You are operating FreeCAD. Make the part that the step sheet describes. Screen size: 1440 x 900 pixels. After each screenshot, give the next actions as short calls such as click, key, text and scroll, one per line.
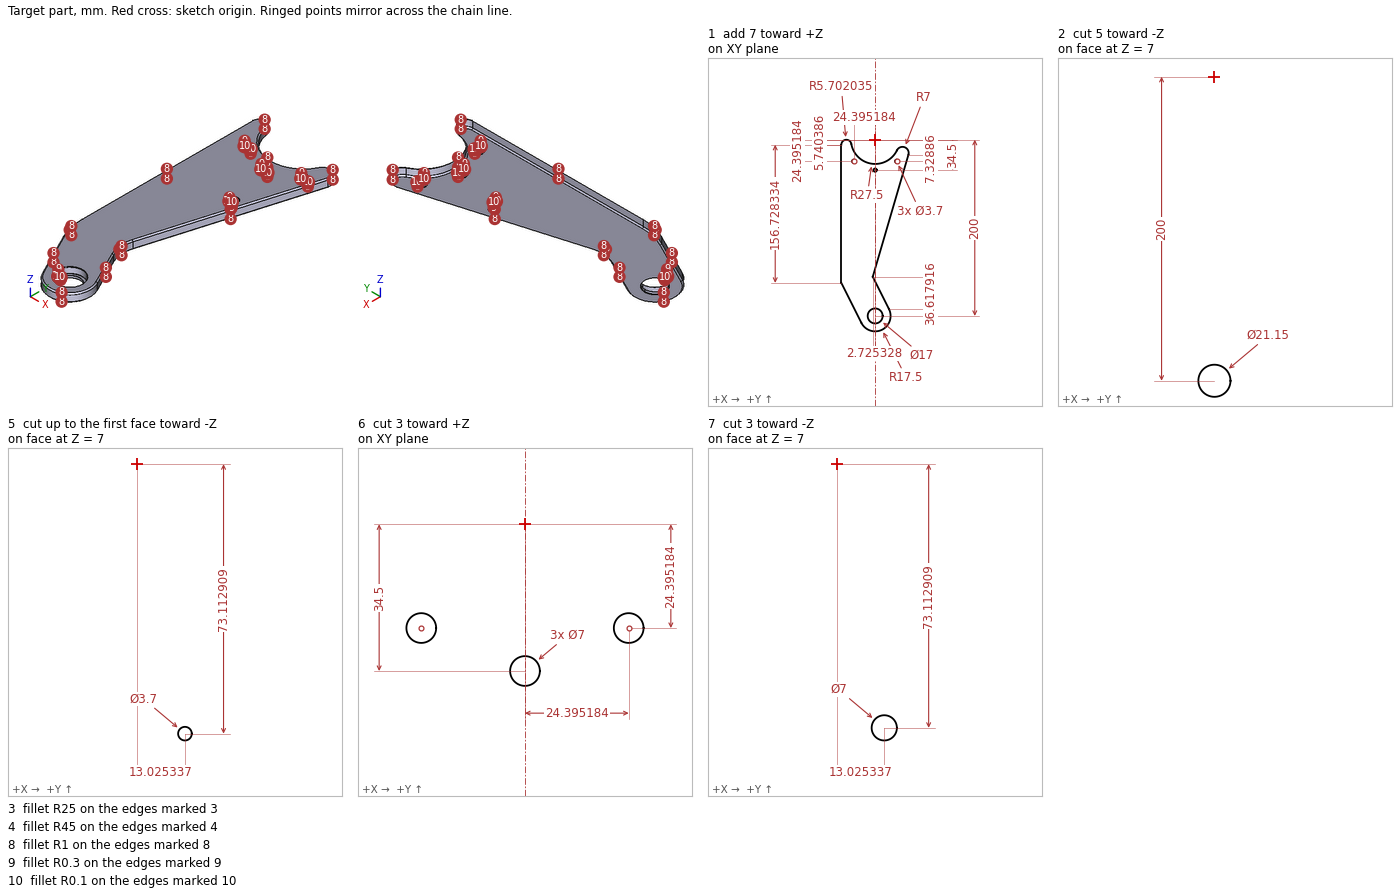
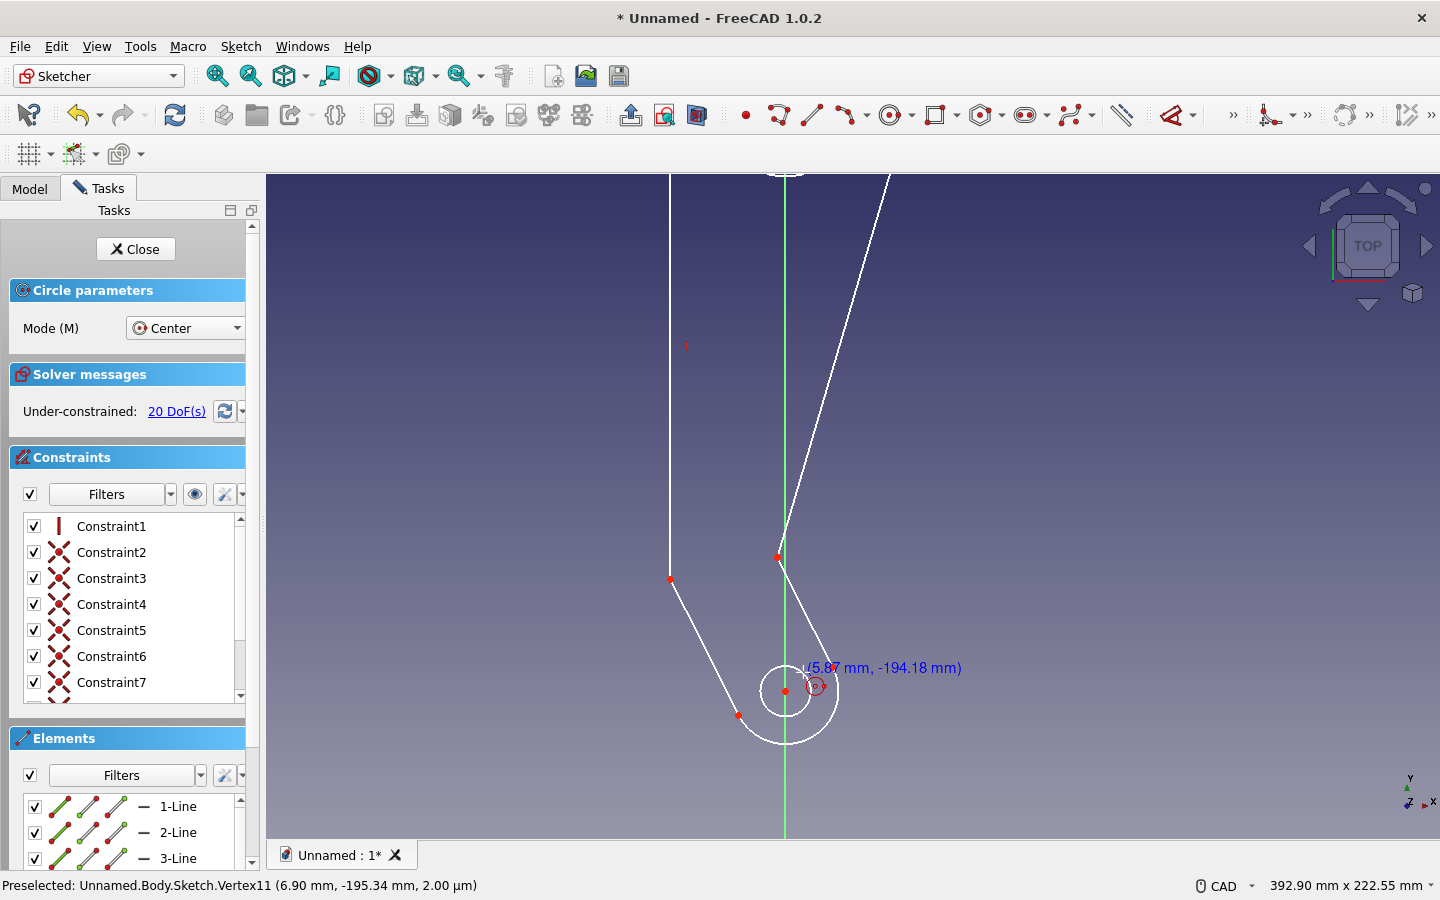
scroll(785, 693, down, 2)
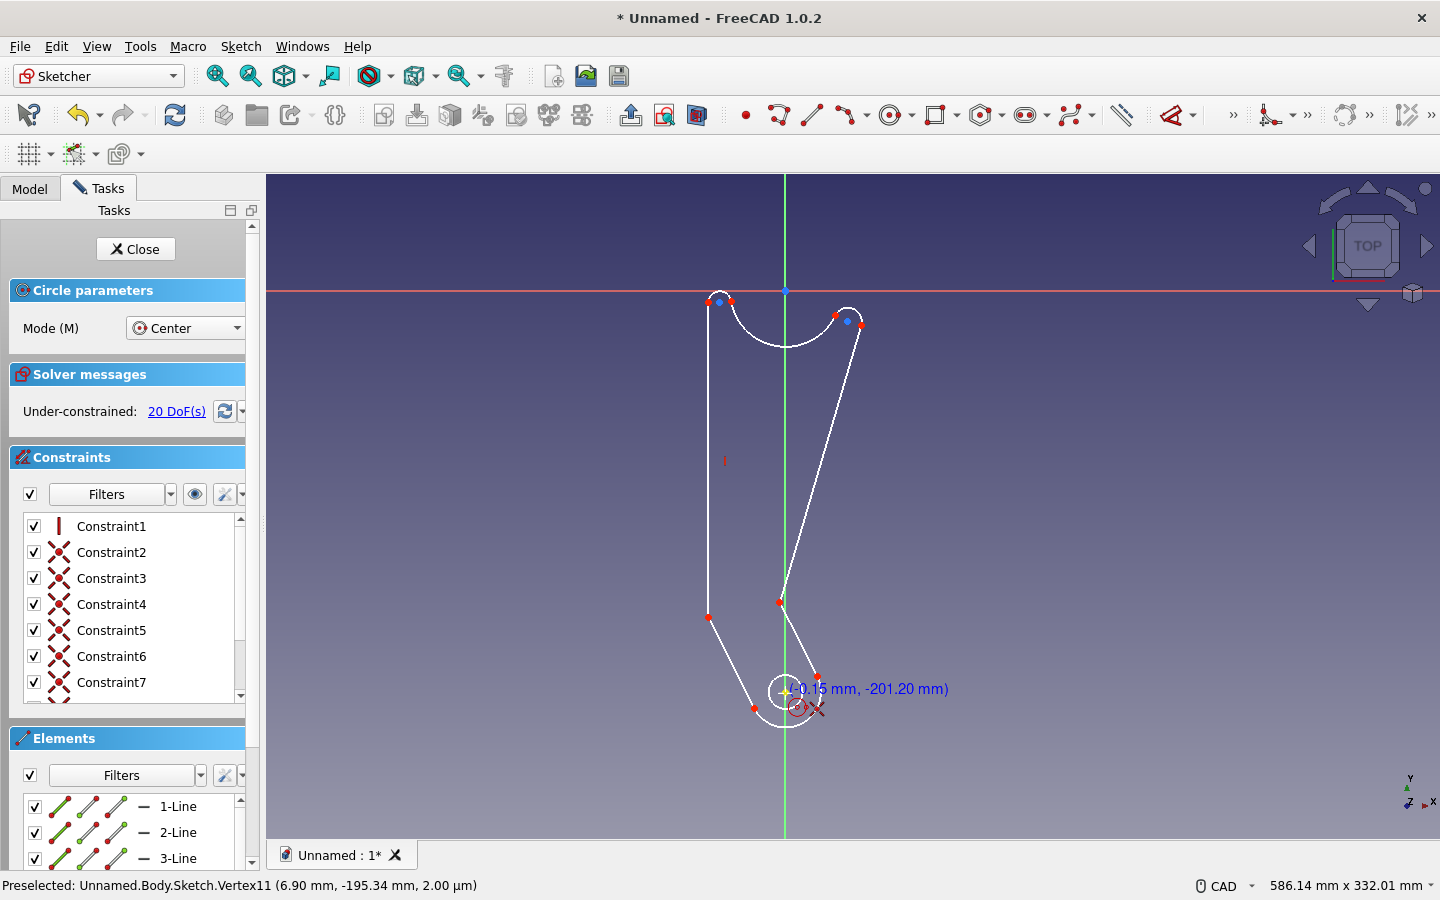
scroll(737, 340, up, 10)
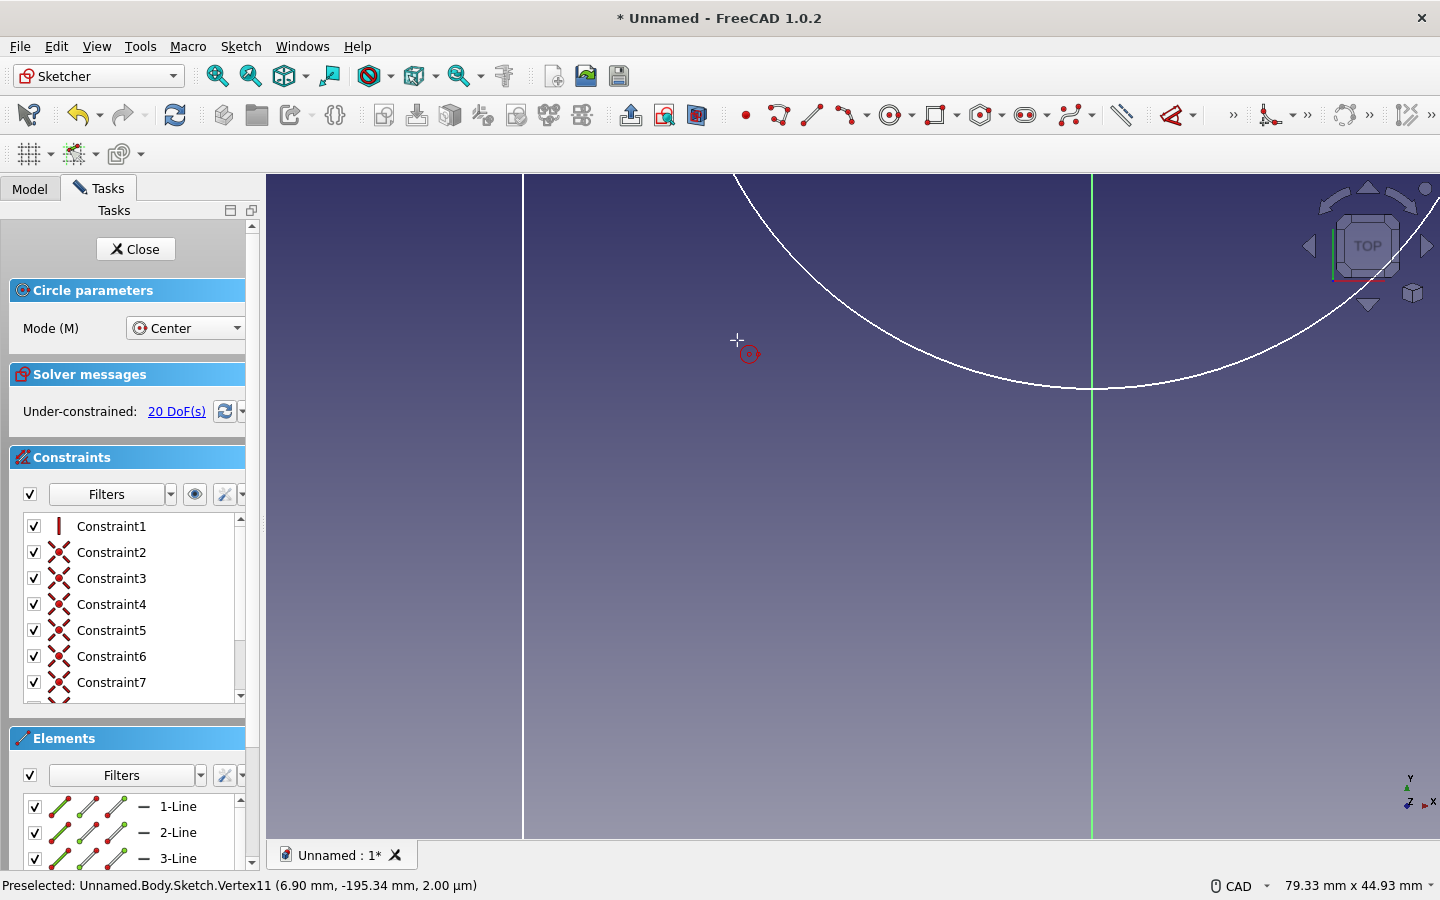
scroll(737, 340, down, 10)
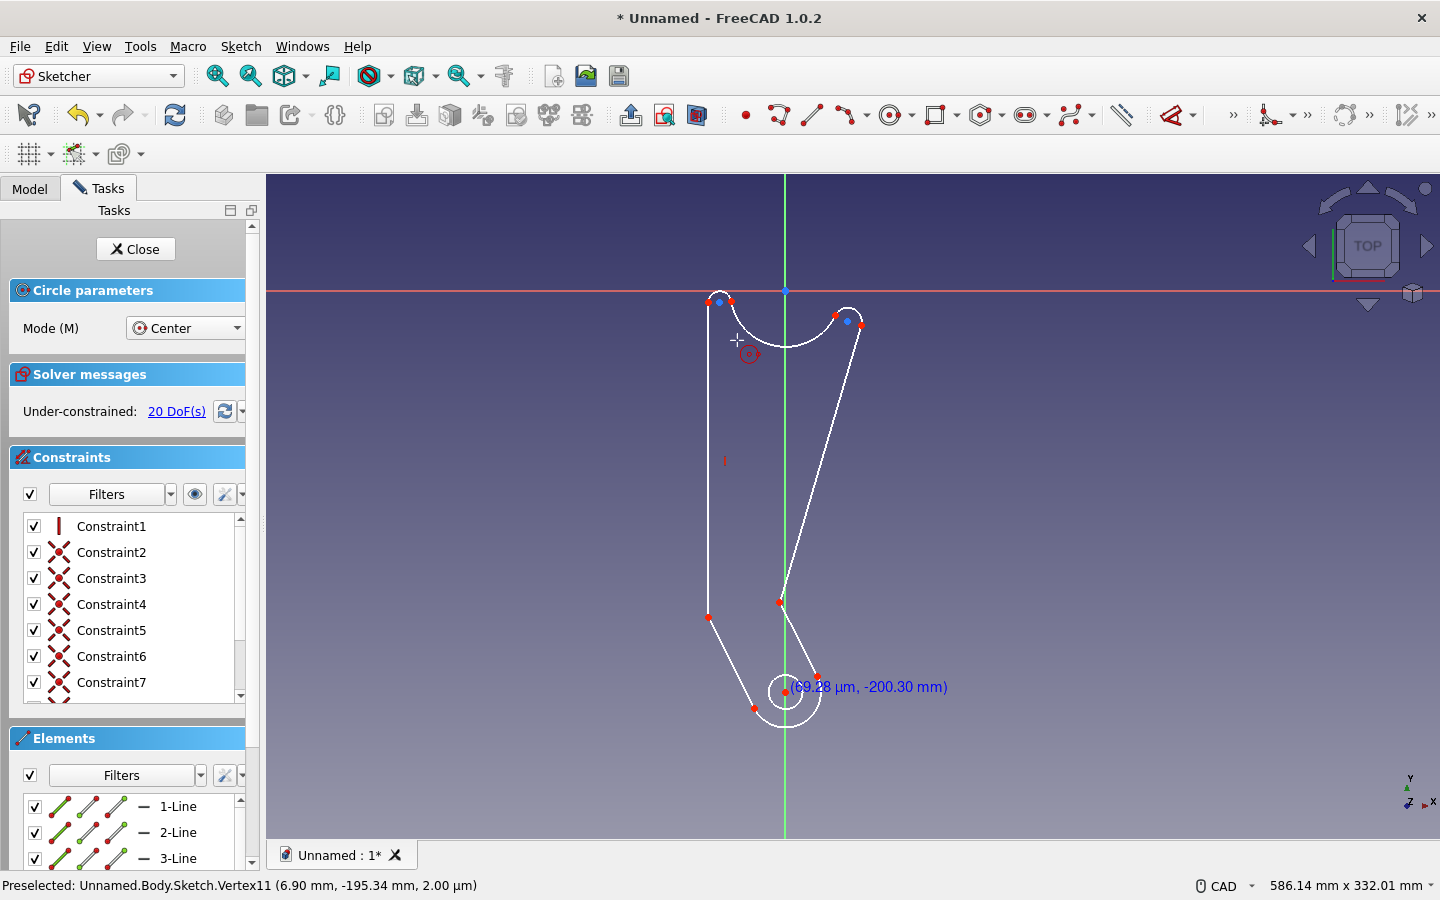
click(737, 340)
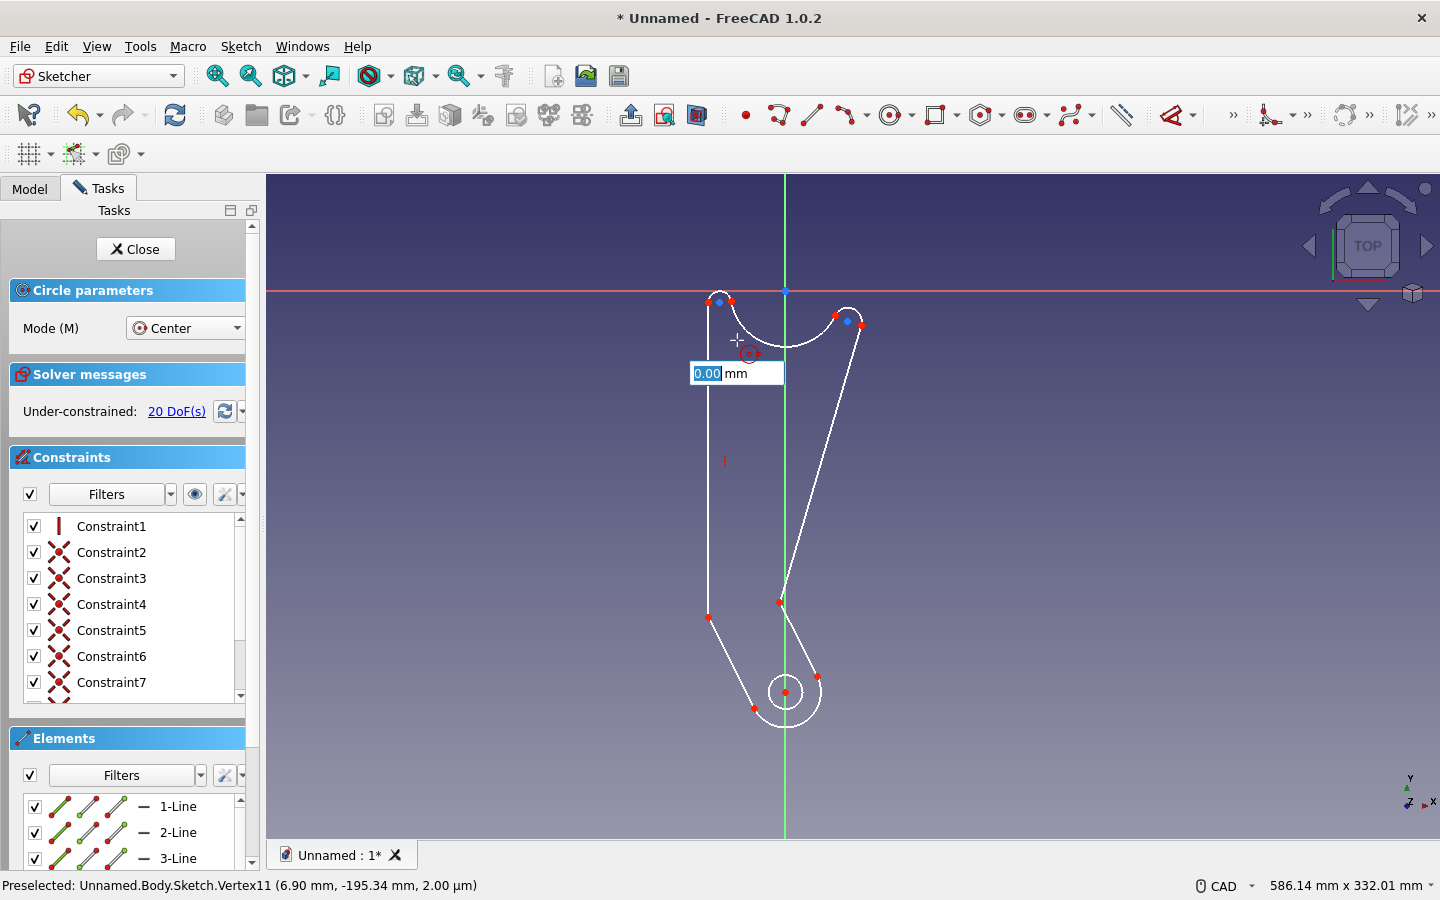
scroll(734, 337, up, 8)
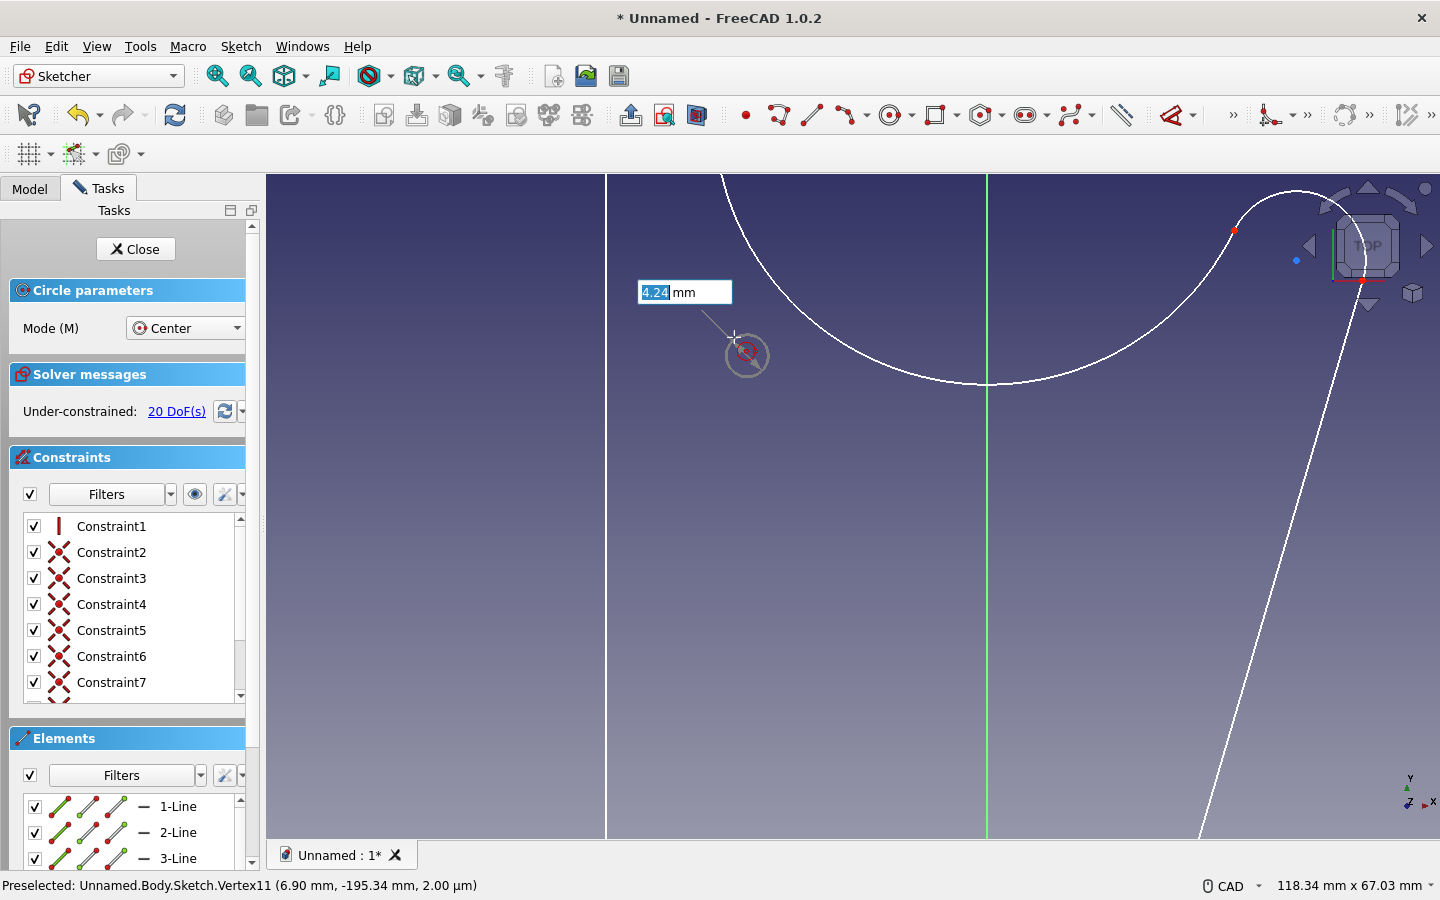
click(732, 337)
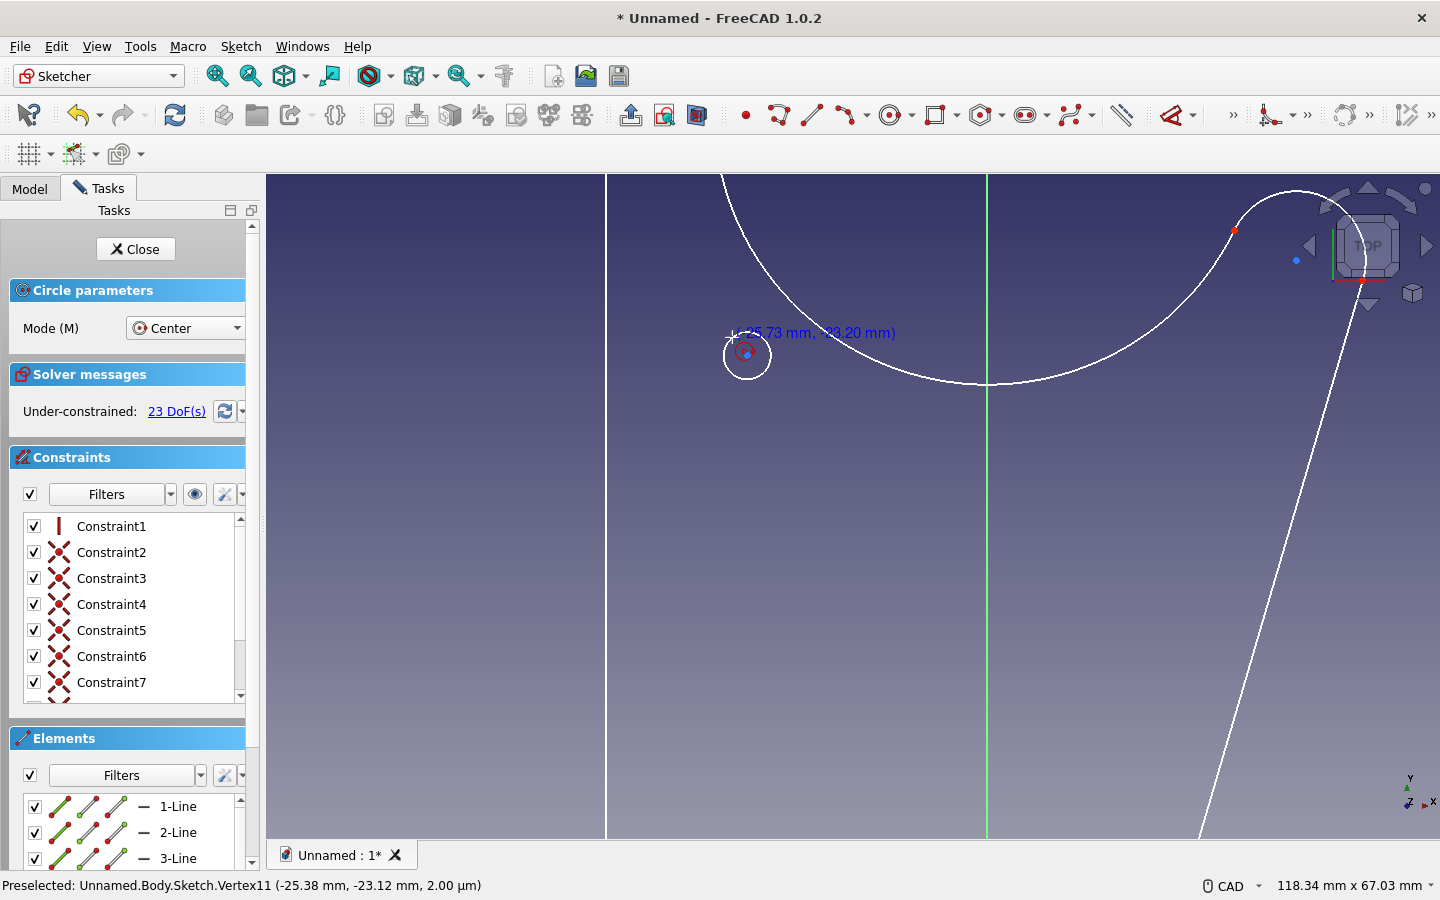
scroll(987, 450, up, 2)